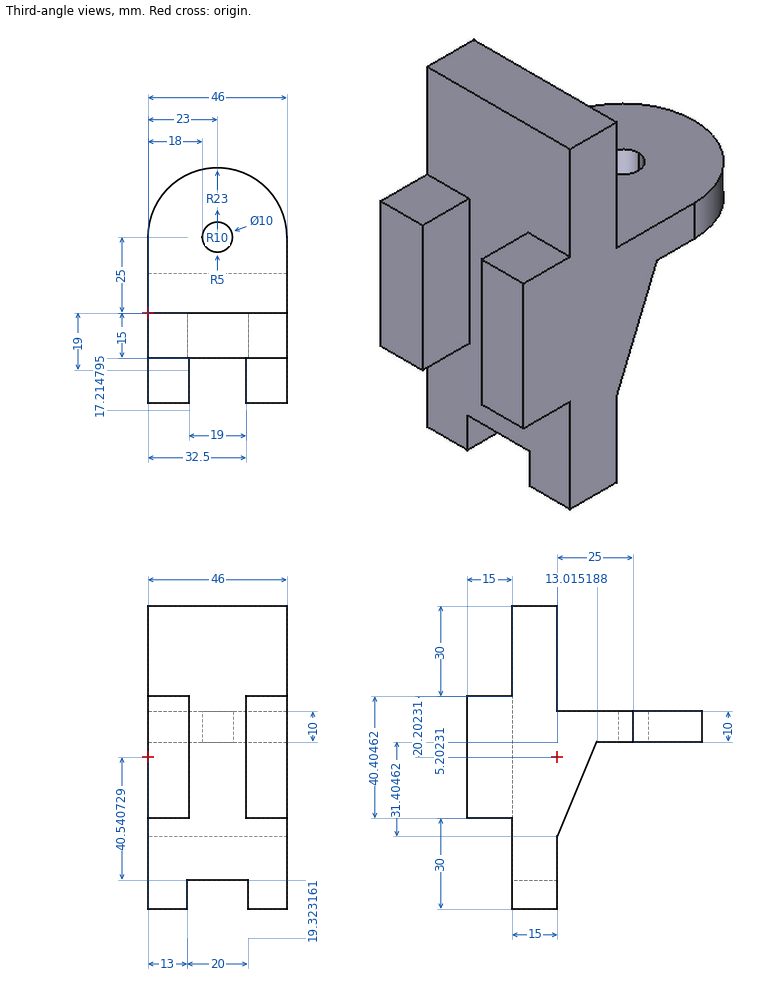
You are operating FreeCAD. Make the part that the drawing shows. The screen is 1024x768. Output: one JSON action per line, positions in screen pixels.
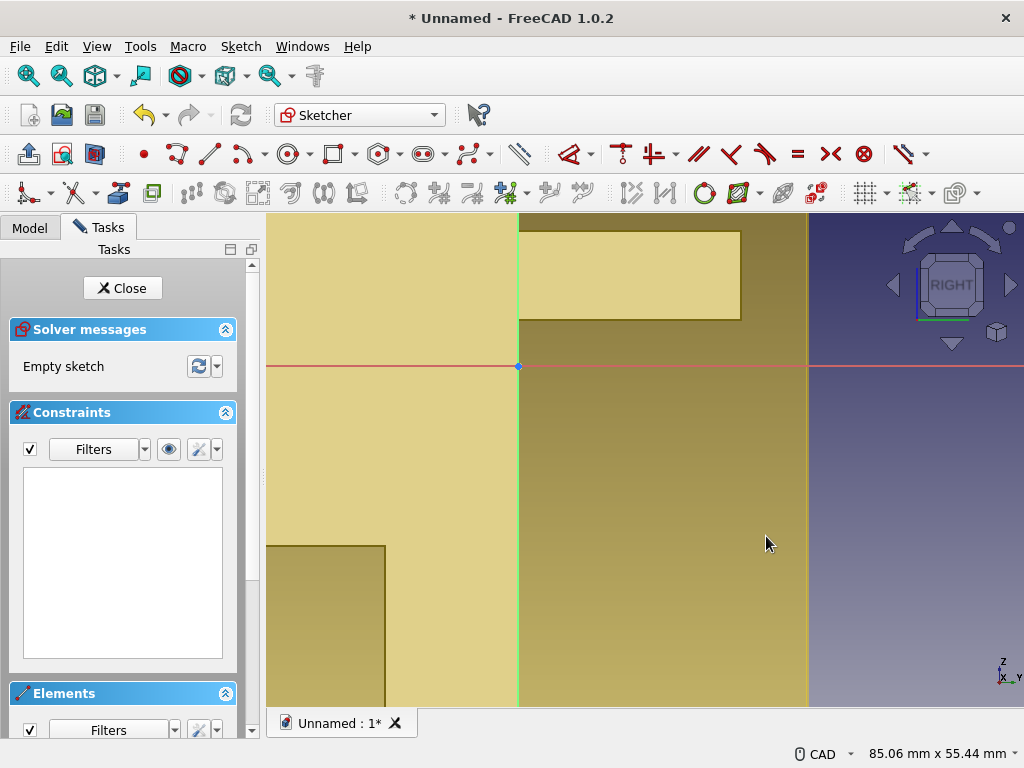
{"action": "left_click", "coordinate": [177, 154]}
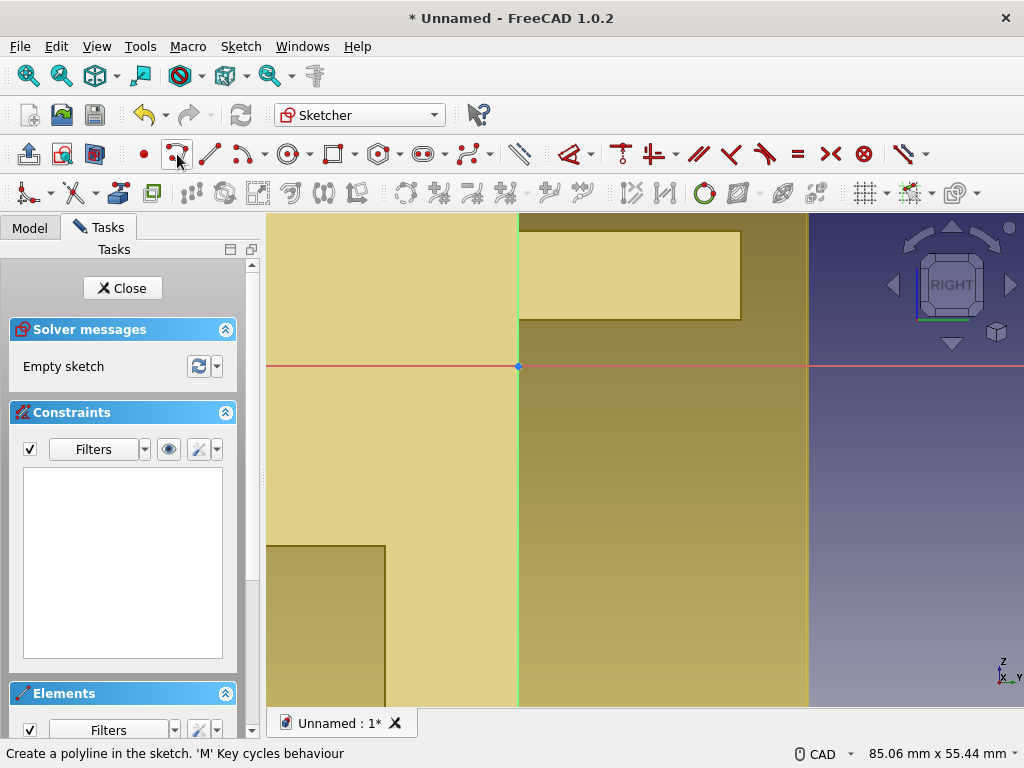
{"action": "left_click", "coordinate": [518, 320]}
{"action": "left_click", "coordinate": [527, 600]}
{"action": "left_click", "coordinate": [634, 320]}
{"action": "left_click", "coordinate": [518, 321]}
{"action": "key", "text": "Escape"}
{"action": "key", "text": "Escape"}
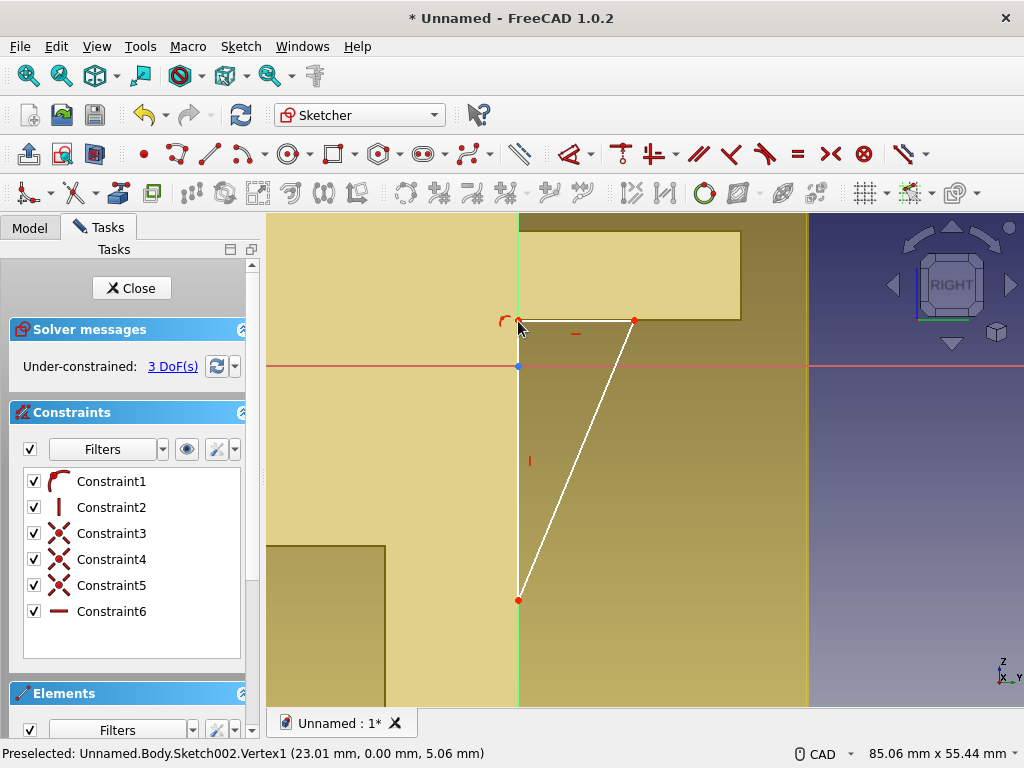
{"action": "left_click", "coordinate": [568, 154]}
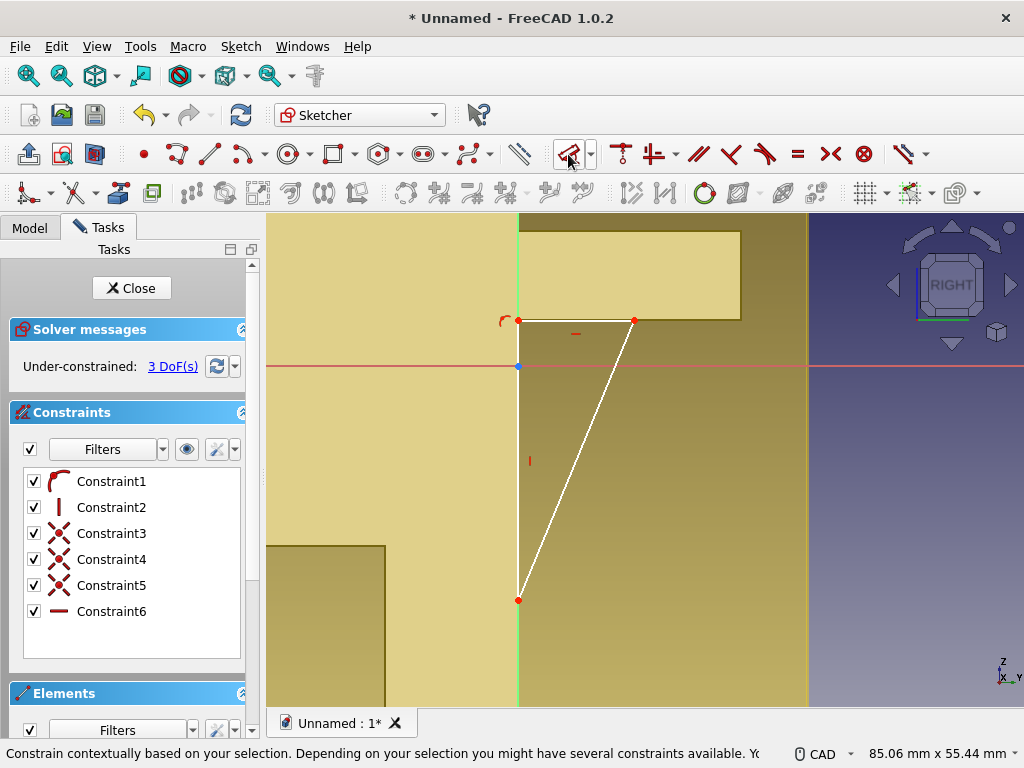
{"action": "left_click", "coordinate": [518, 405]}
{"action": "left_click", "coordinate": [484, 461]}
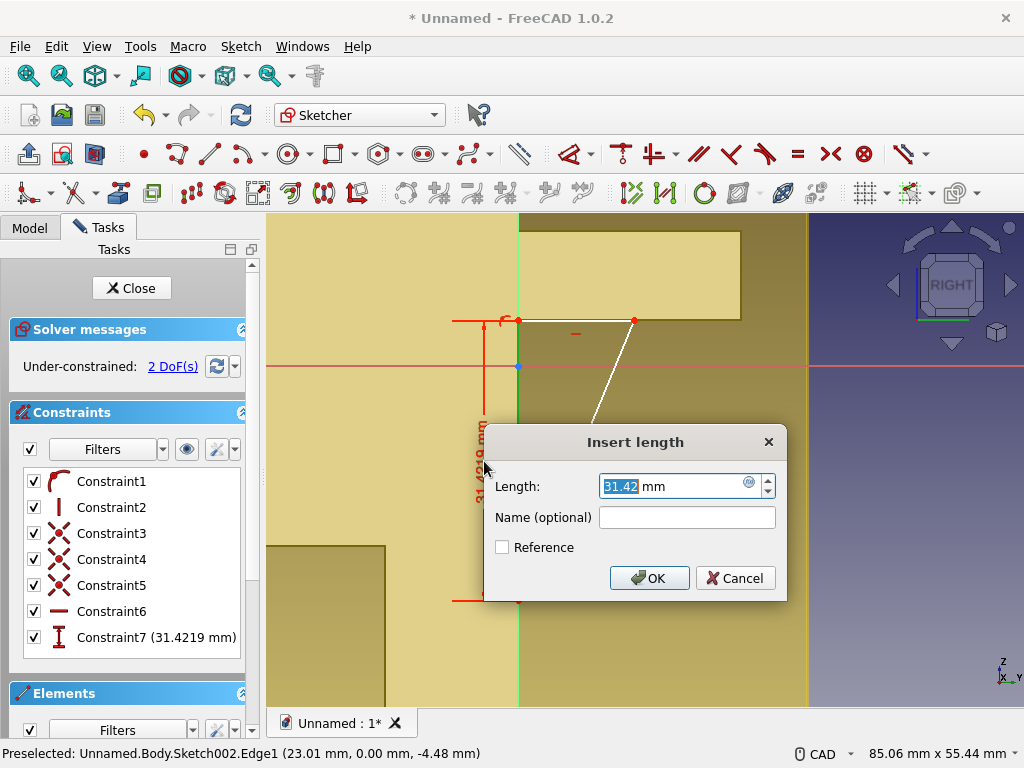
{"action": "type", "text": "31.40462"}
{"action": "key", "text": "Return"}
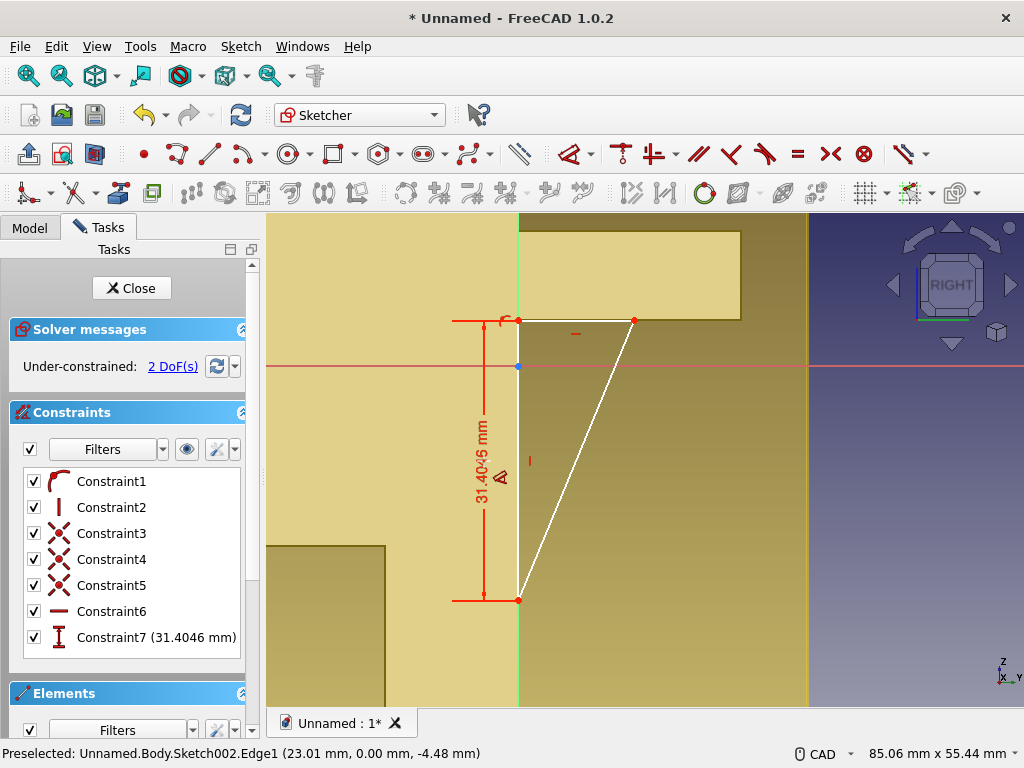
{"action": "left_click", "coordinate": [518, 321]}
{"action": "left_click", "coordinate": [484, 344]}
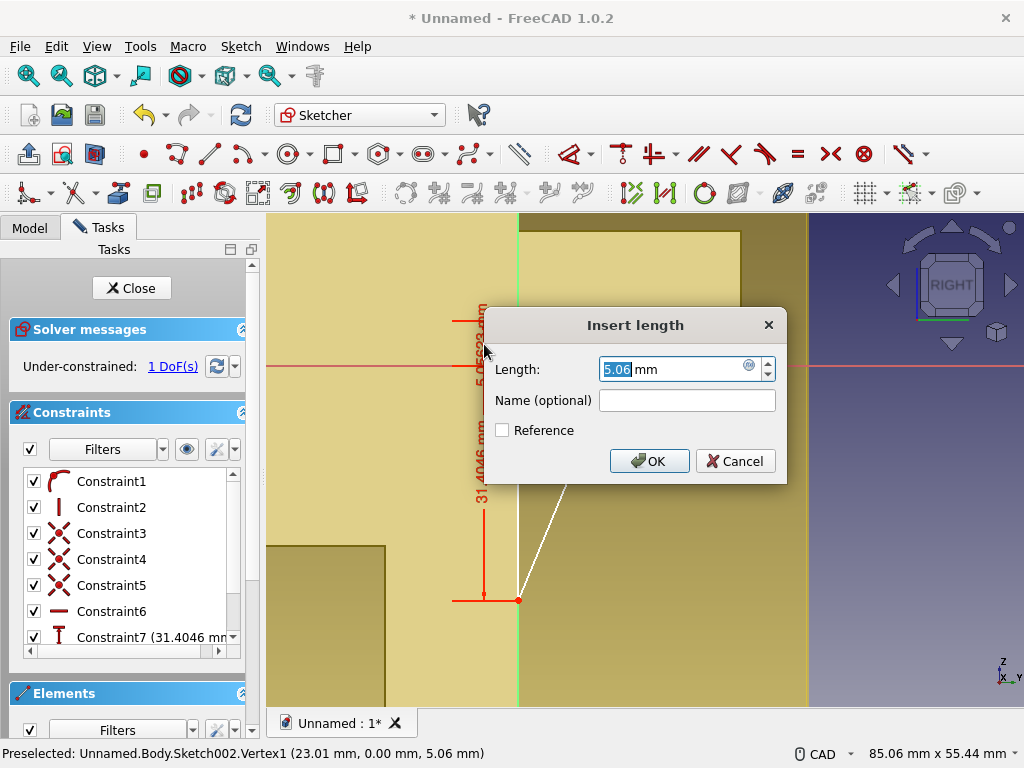
{"action": "type", "text": "5.20231"}
{"action": "key", "text": "Return"}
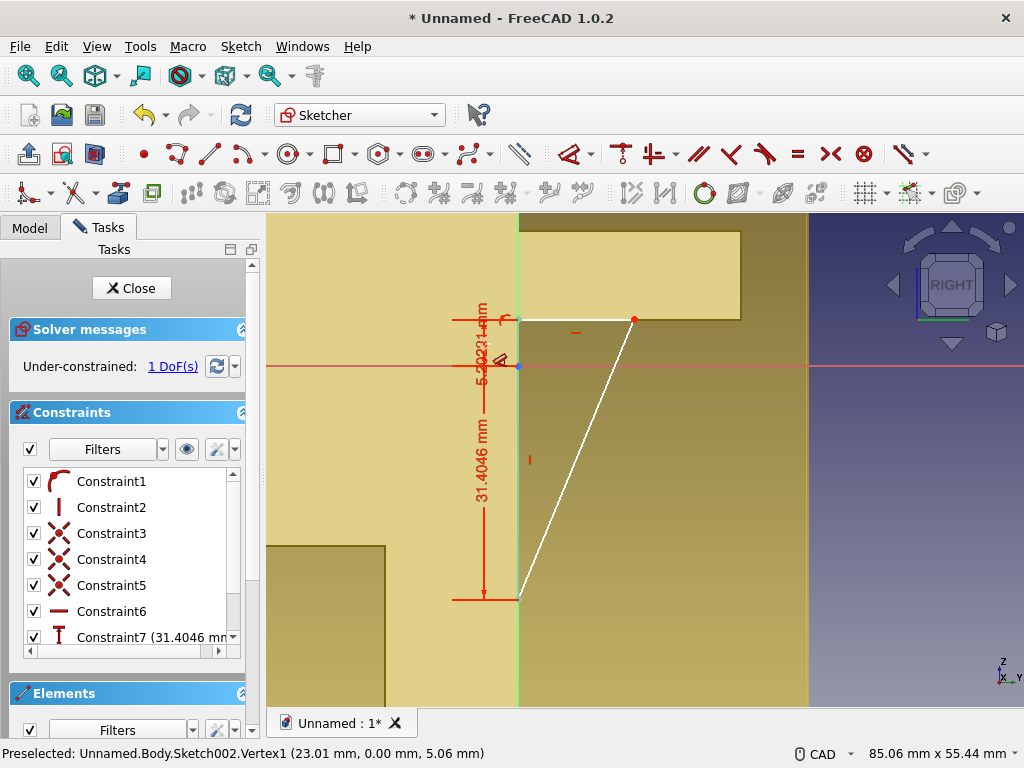
{"action": "left_click", "coordinate": [599, 320]}
{"action": "left_click", "coordinate": [576, 286]}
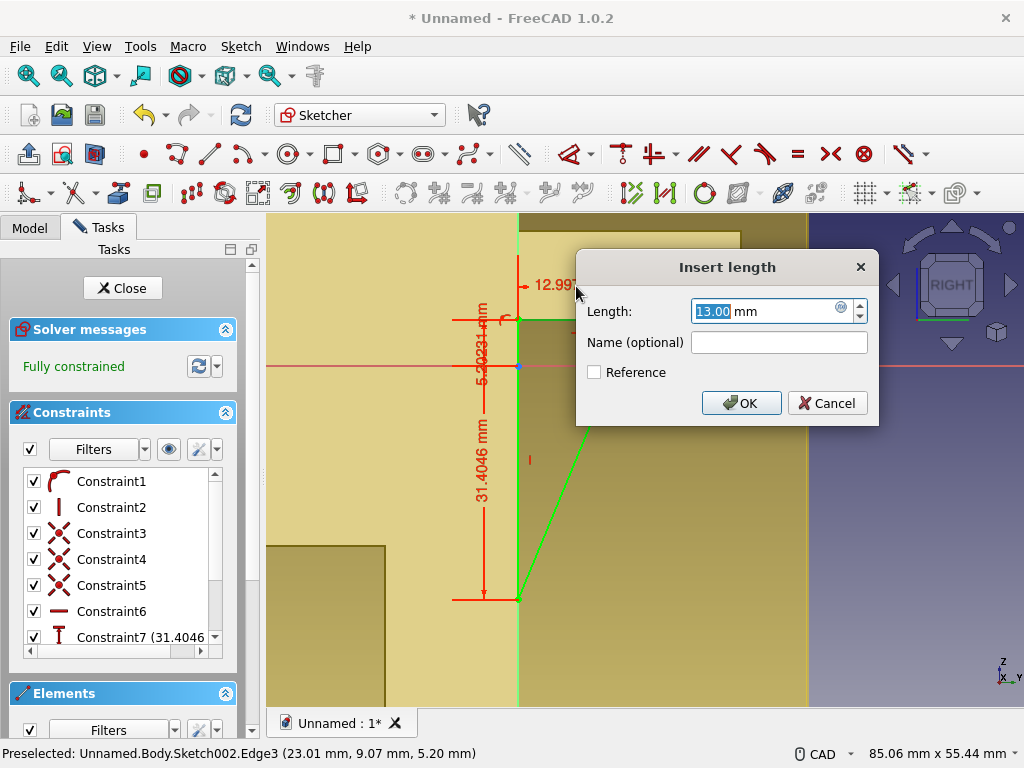
{"action": "type", "text": "13.015188"}
{"action": "key", "text": "Return"}
{"action": "key", "text": "Escape"}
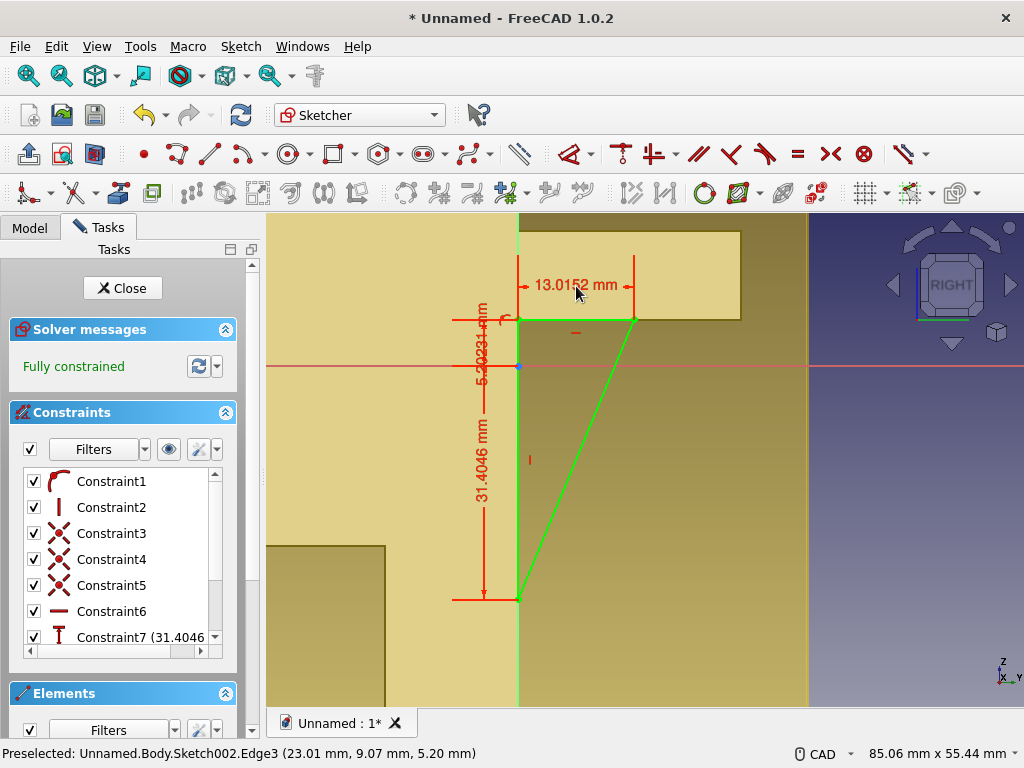
{"action": "left_click", "coordinate": [123, 288]}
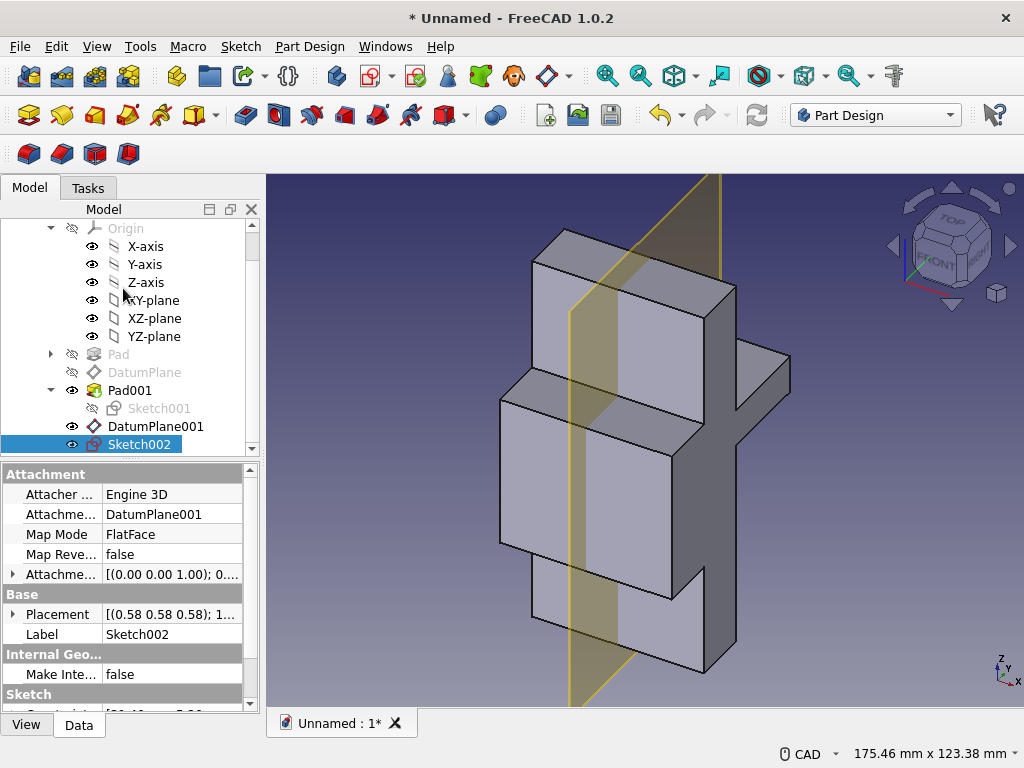
{"action": "left_click", "coordinate": [29, 116]}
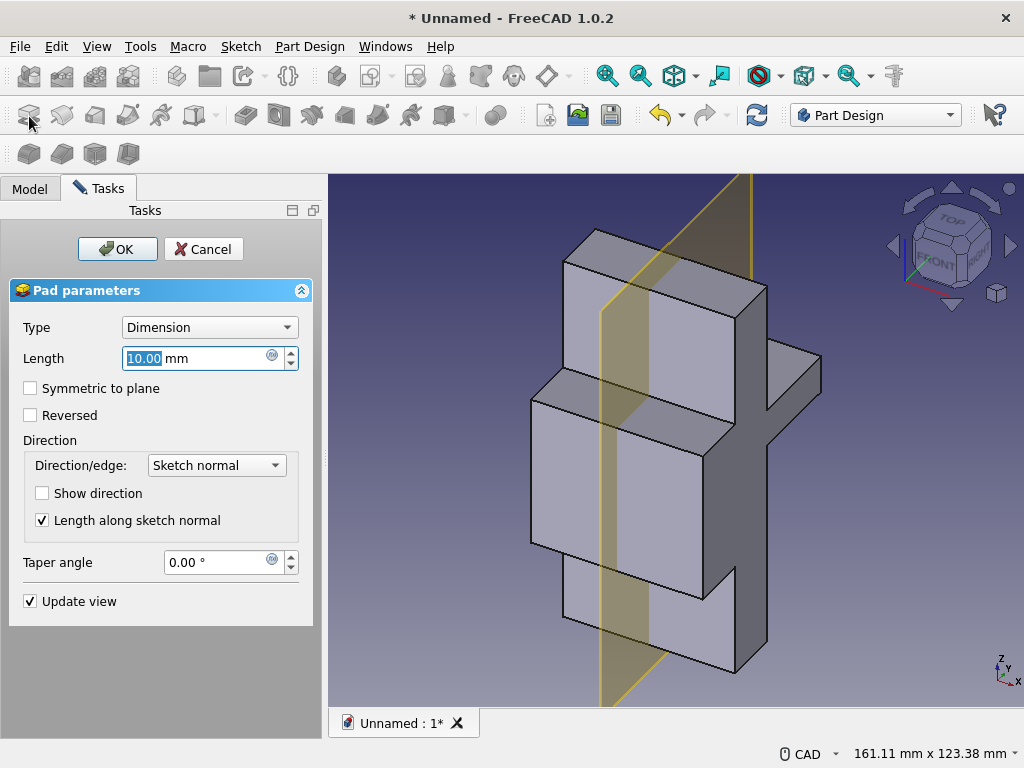
{"action": "type", "text": "46"}
{"action": "key", "text": "Tab"}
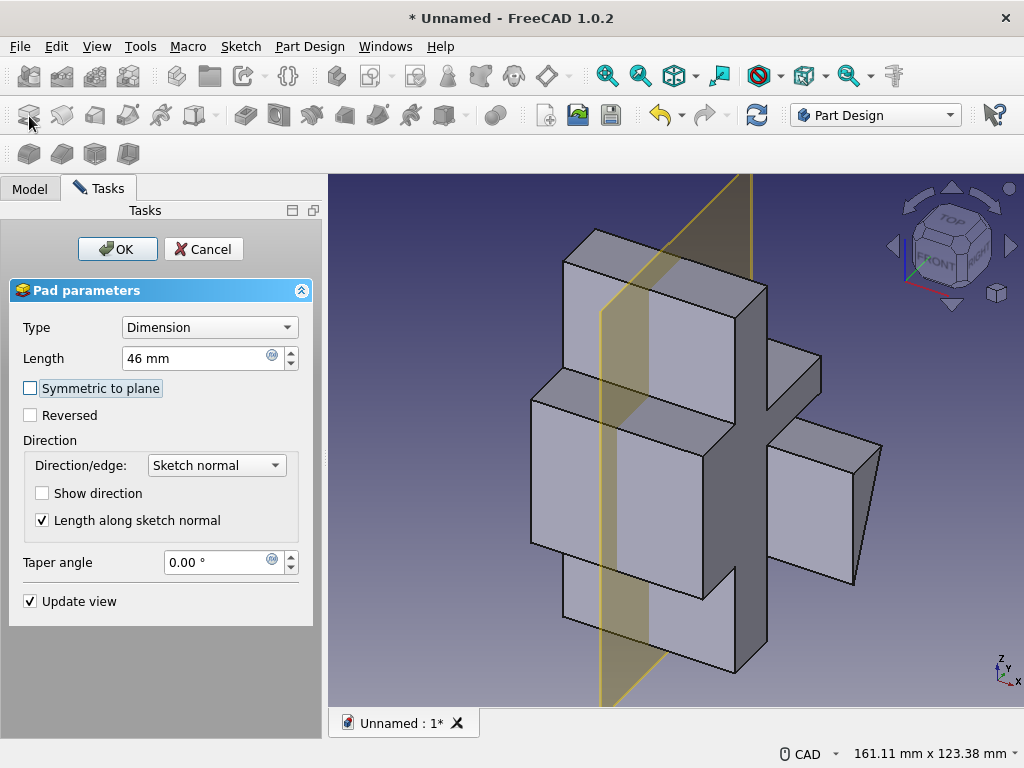
{"action": "left_click", "coordinate": [31, 388]}